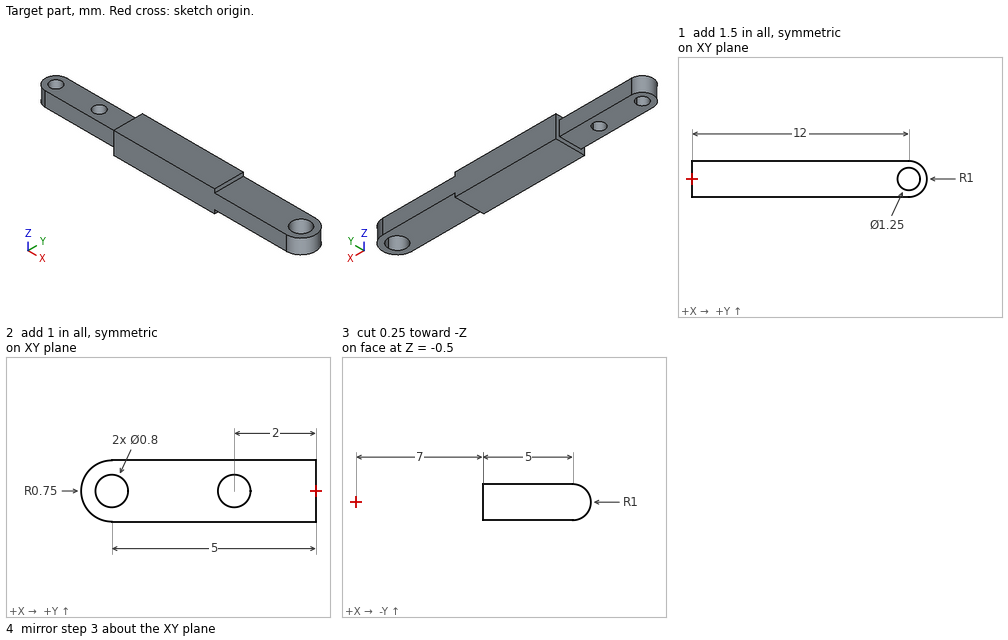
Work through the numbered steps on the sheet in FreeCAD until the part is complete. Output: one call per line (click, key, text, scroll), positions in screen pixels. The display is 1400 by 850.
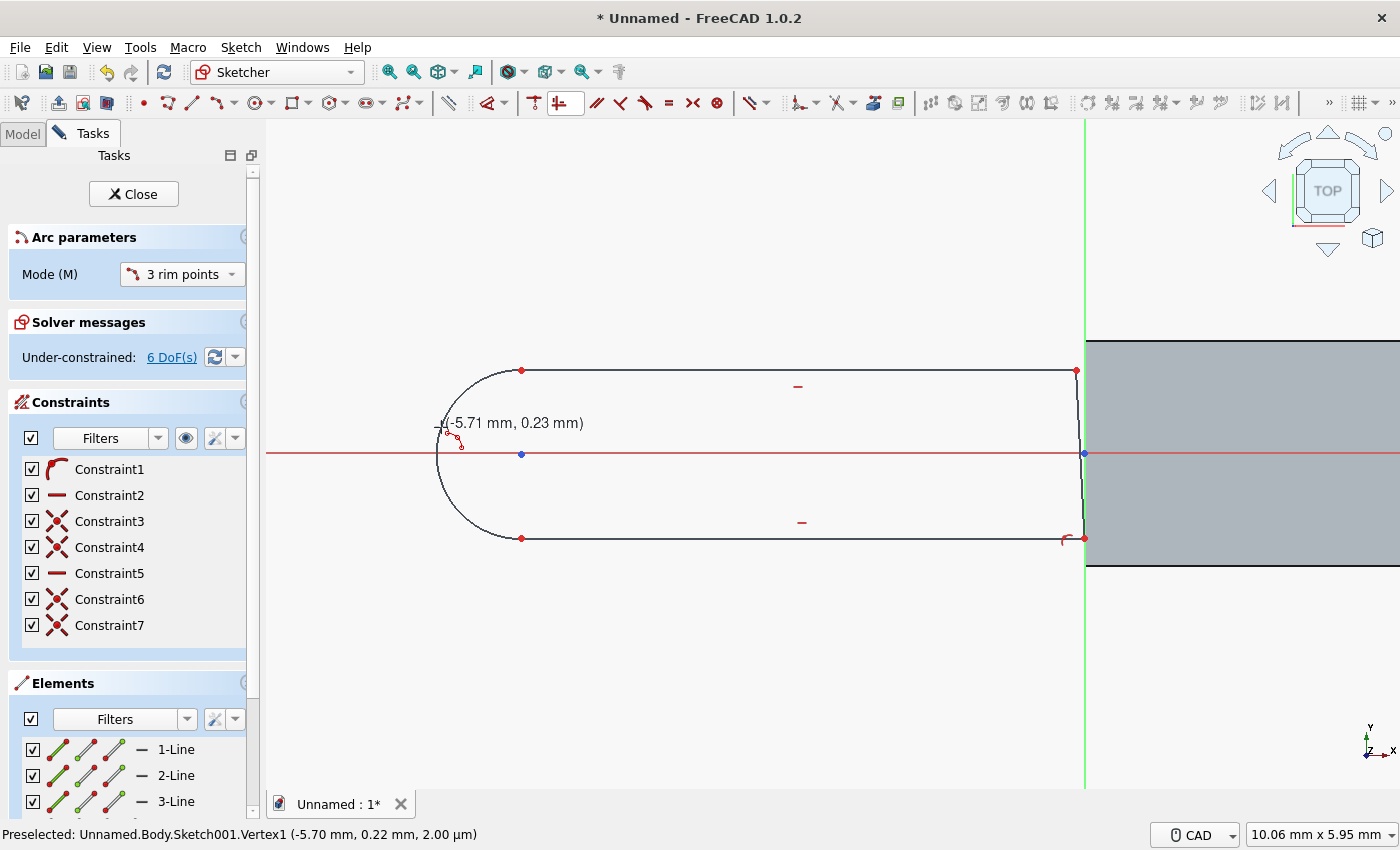
click(256, 104)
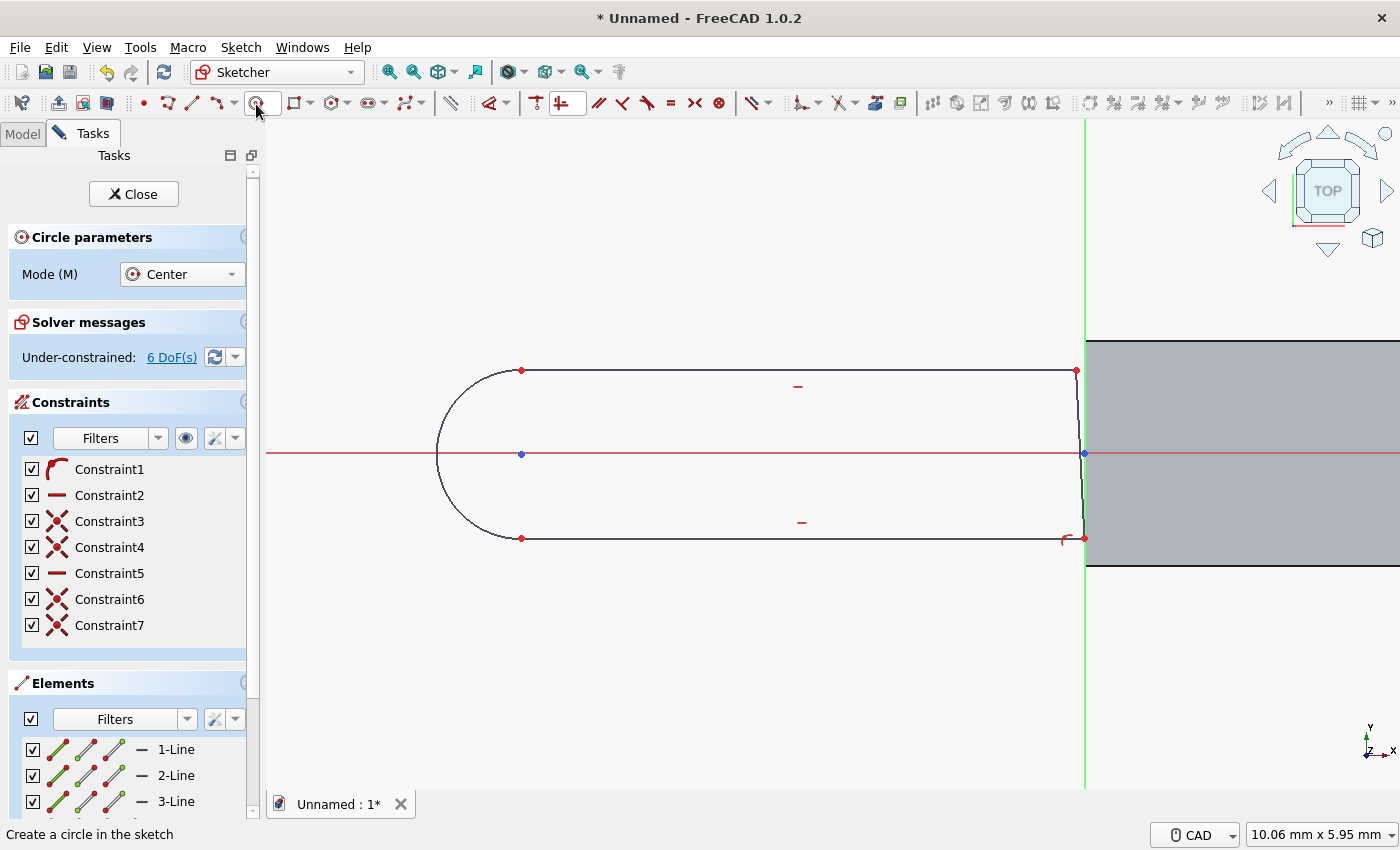
click(859, 453)
move(891, 422)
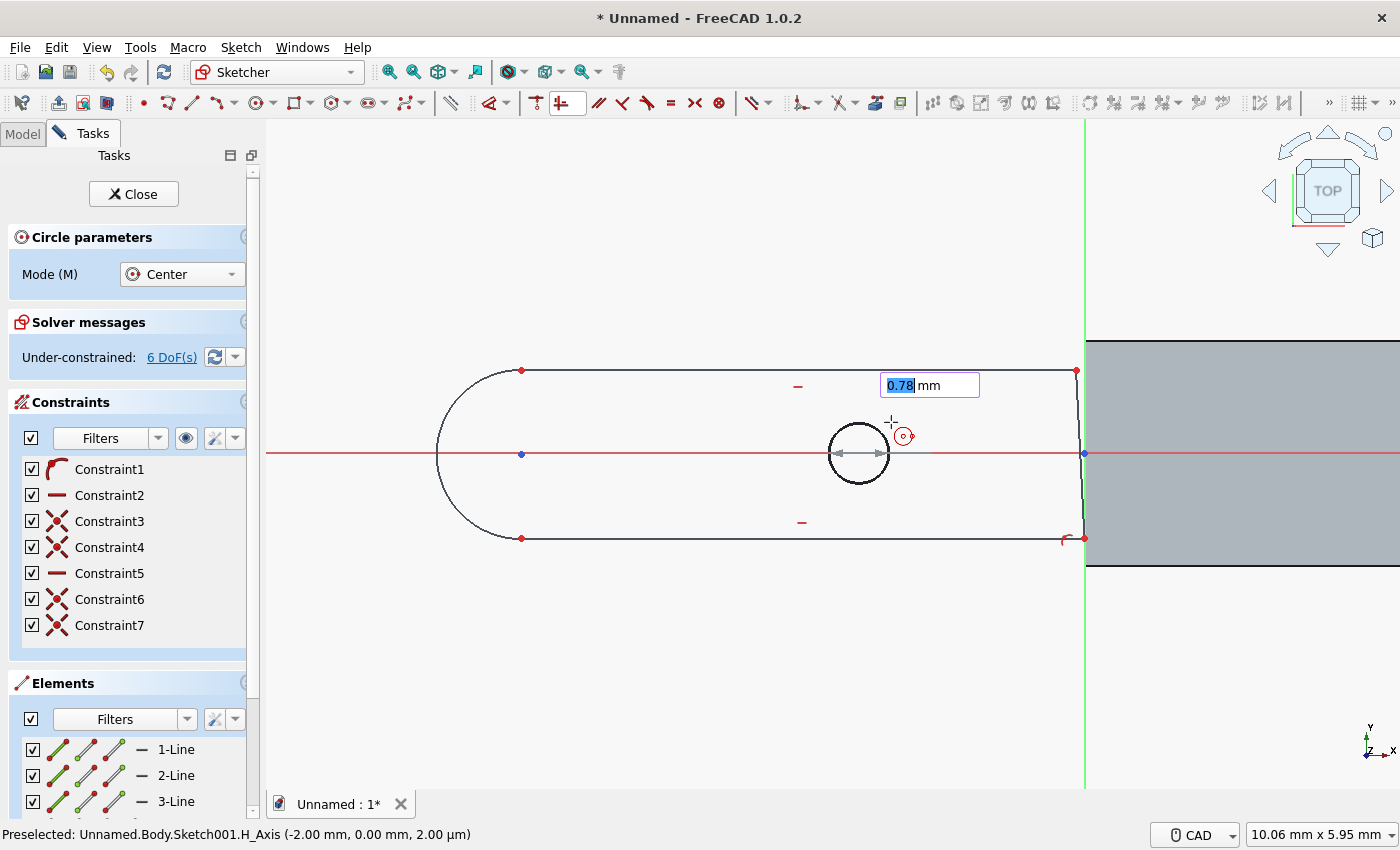
text(0.8)
key(Return)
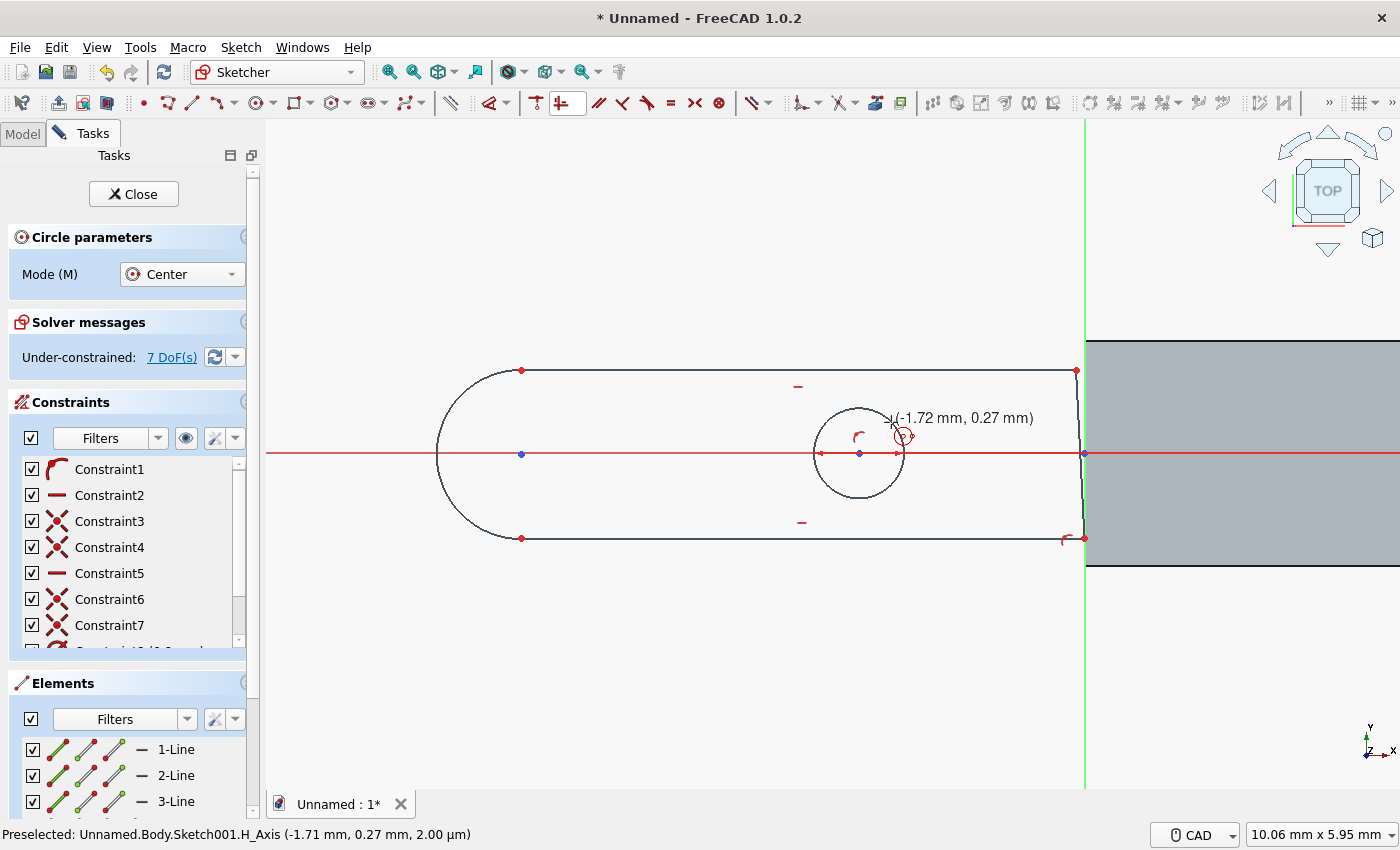
click(521, 453)
move(553, 422)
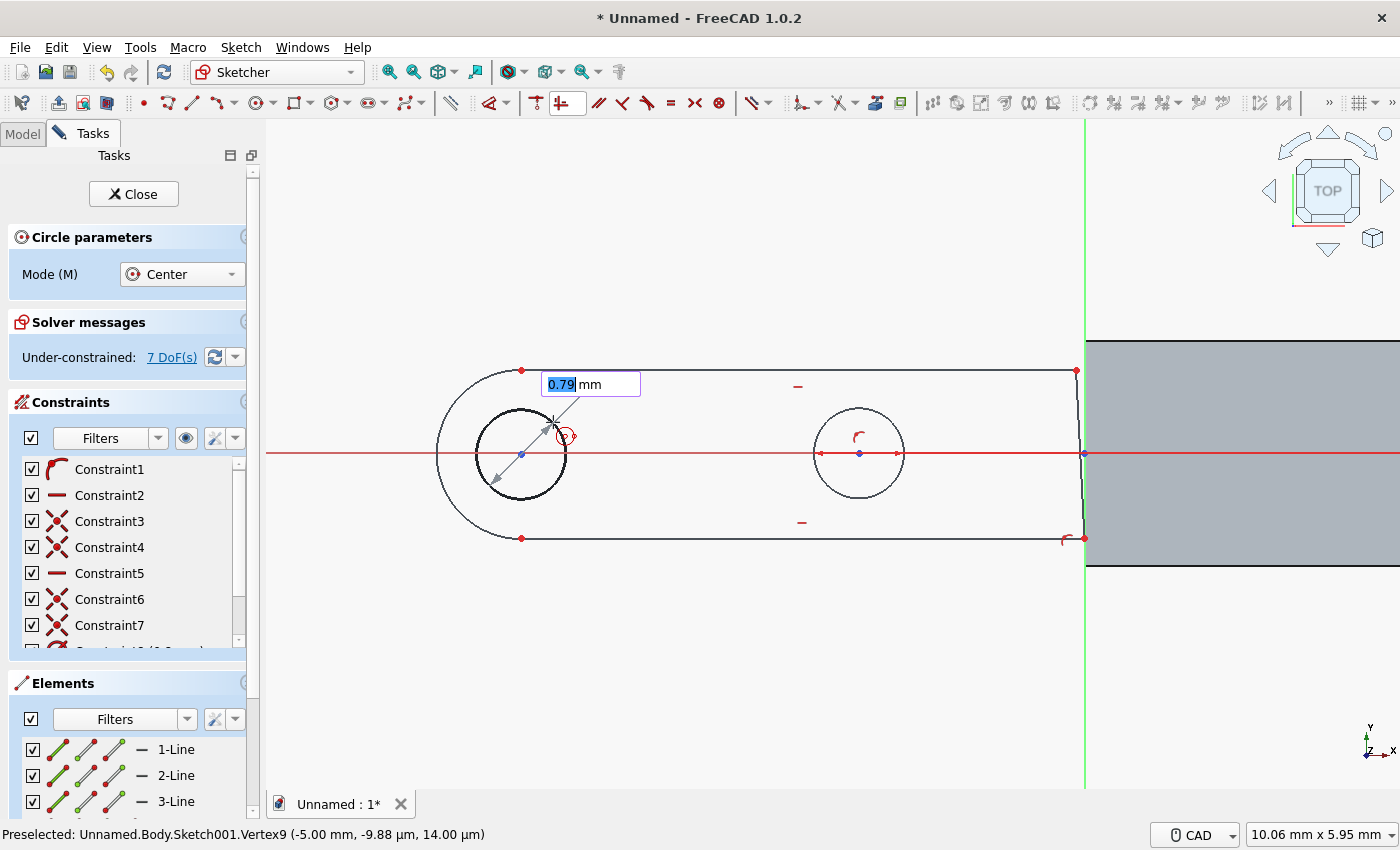
text(0.8)
key(Return)
key(Escape)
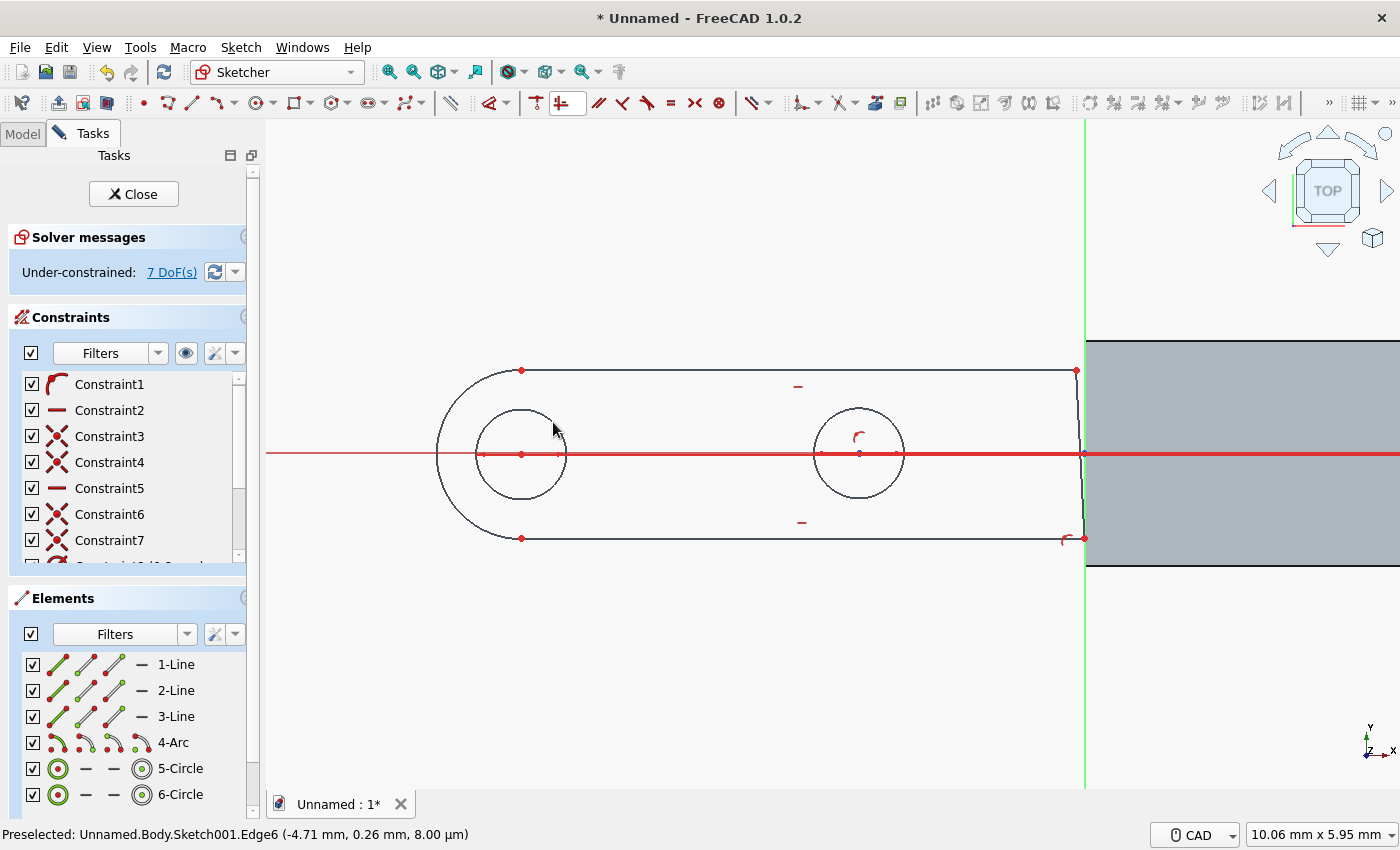
click(690, 539)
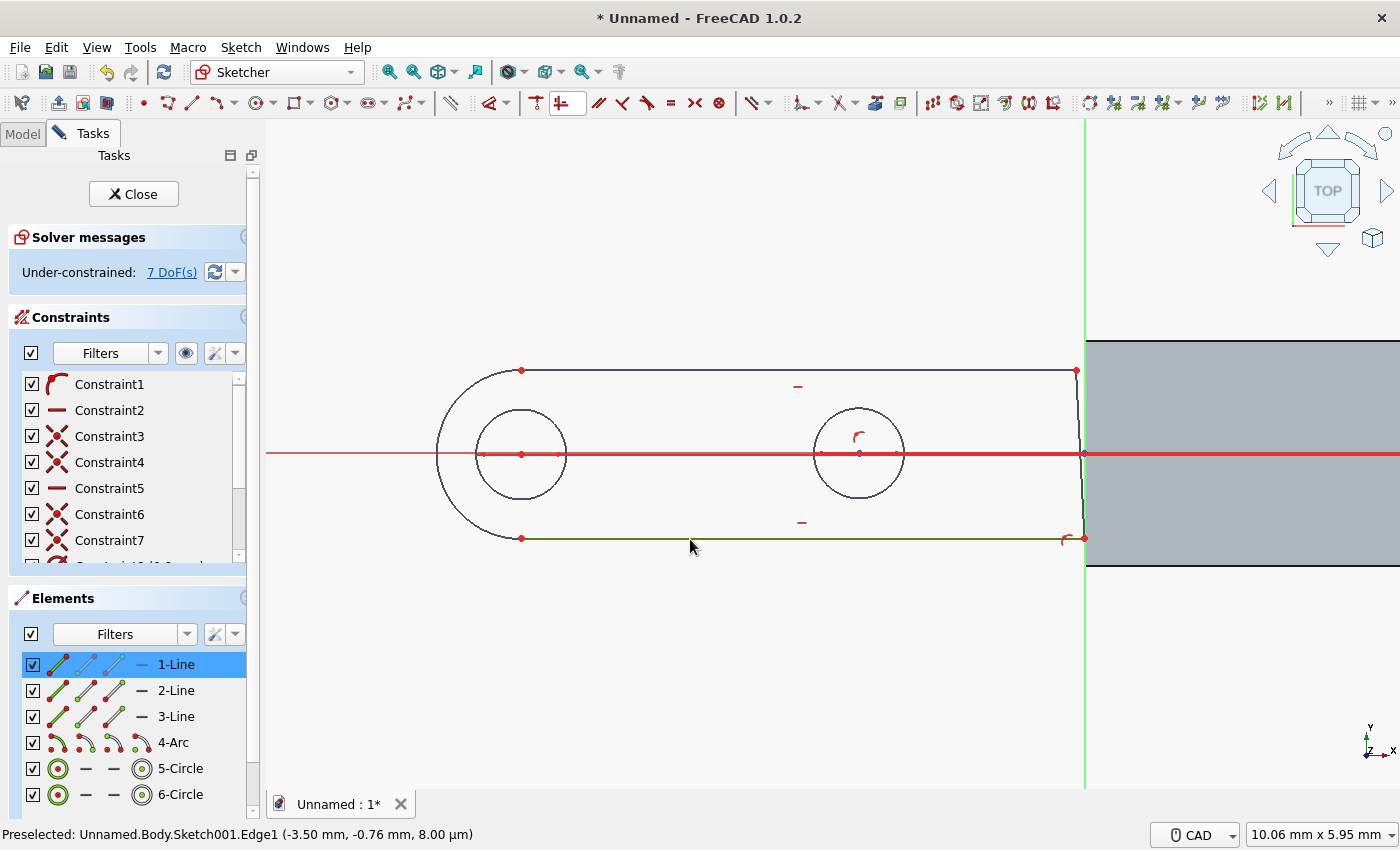
click(453, 405)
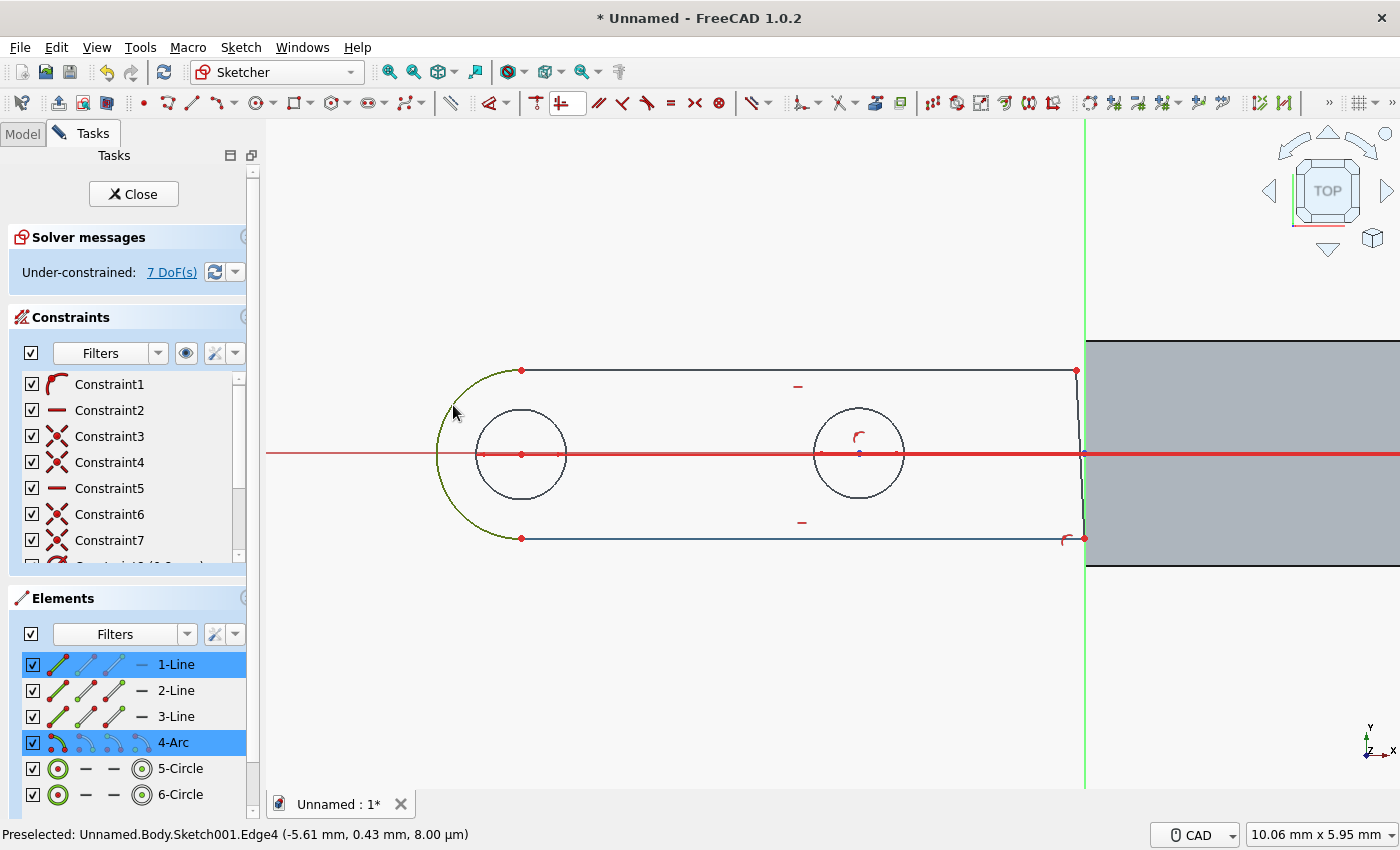
key(t)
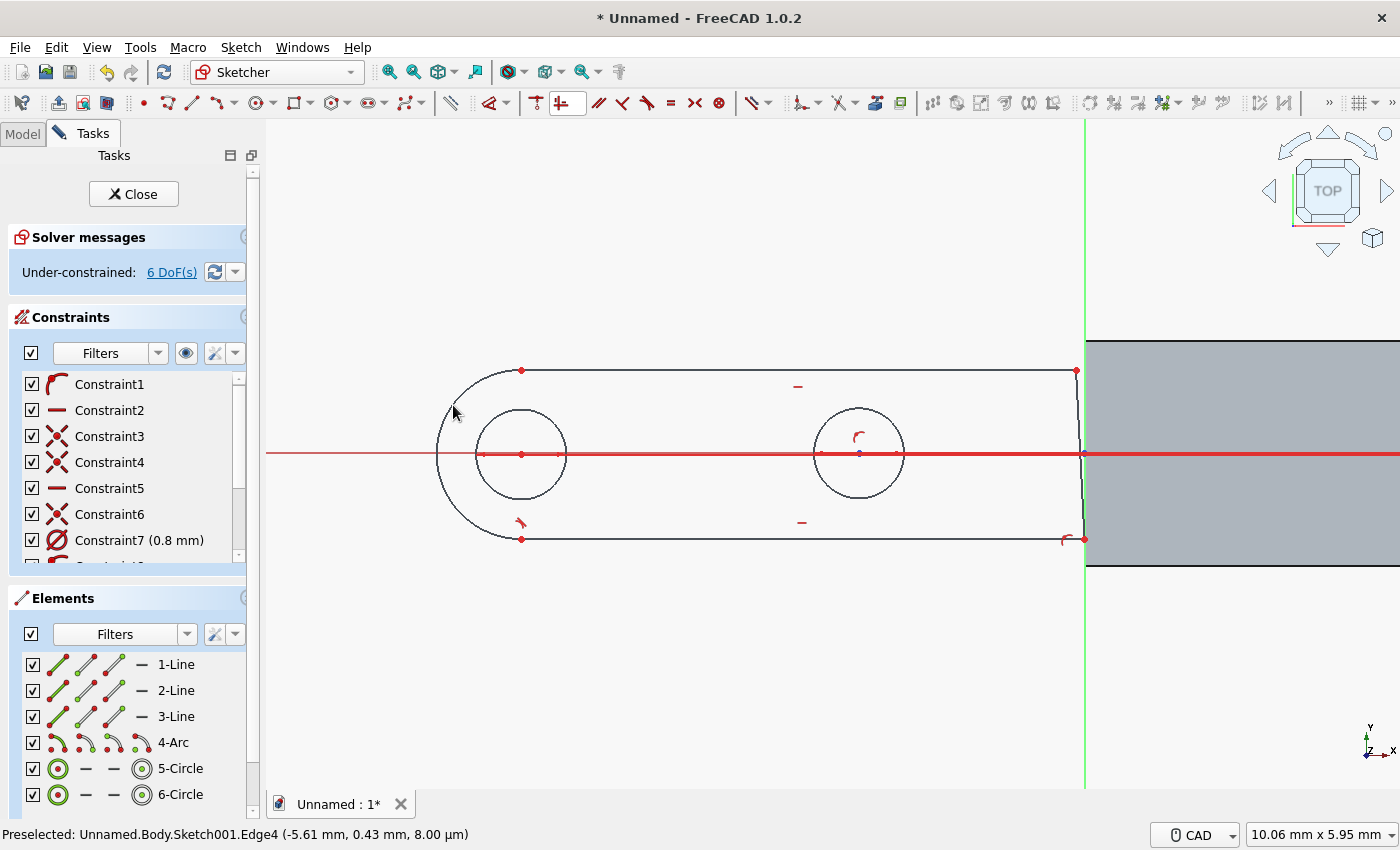
click(910, 370)